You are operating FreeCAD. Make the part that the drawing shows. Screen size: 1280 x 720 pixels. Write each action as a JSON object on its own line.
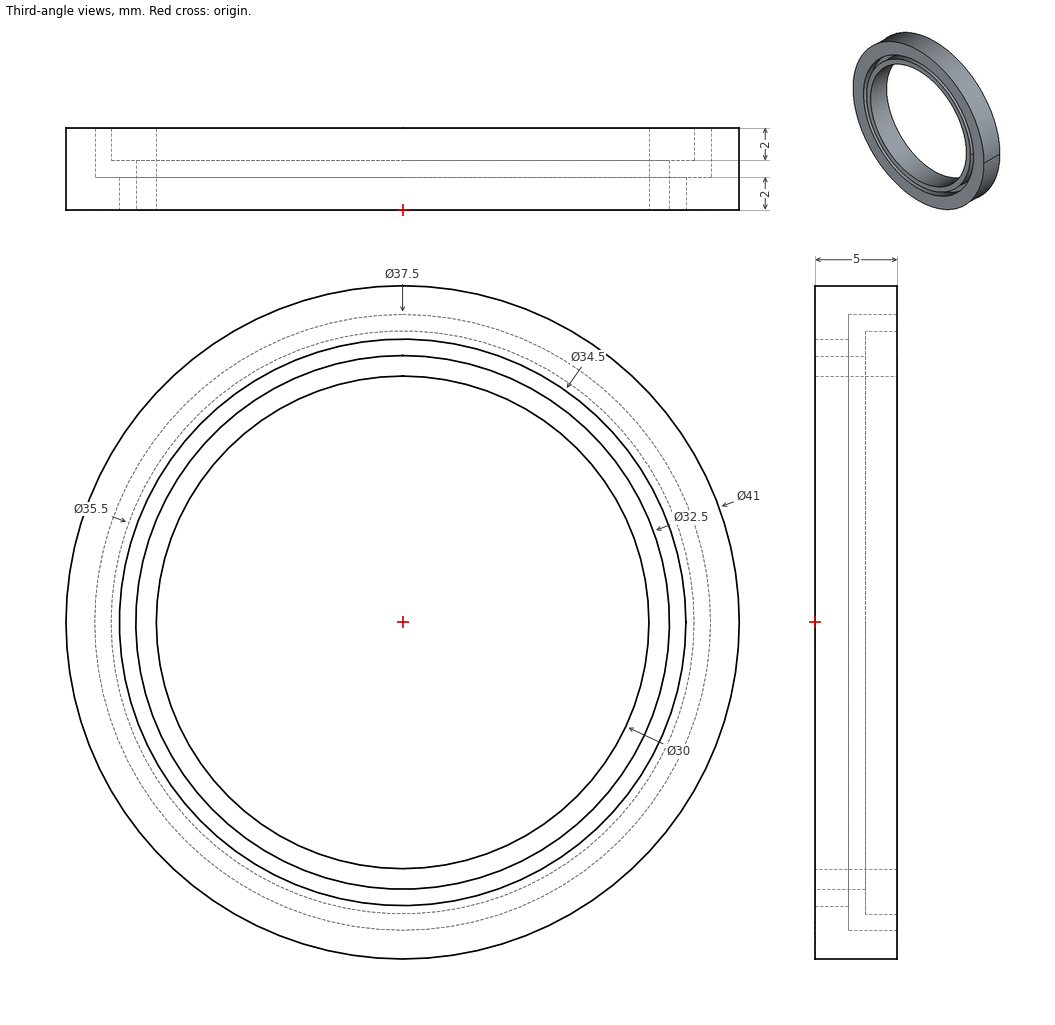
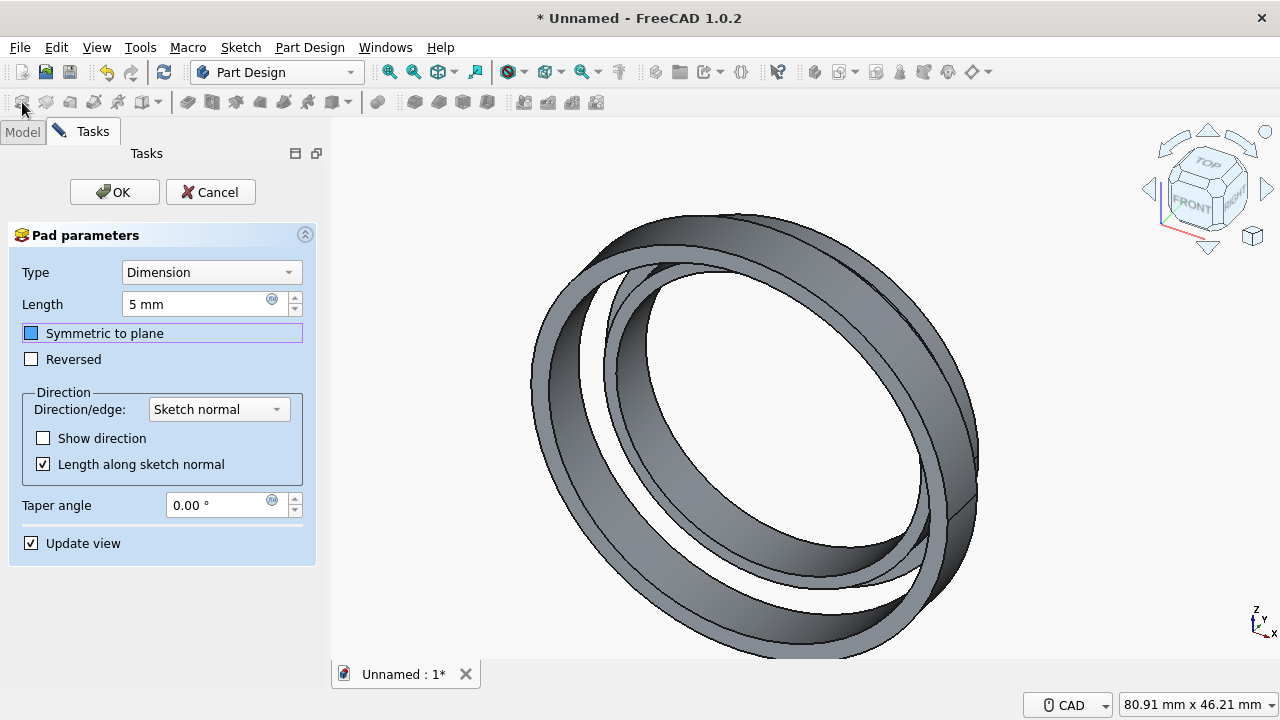
{"action": "left_click", "coordinate": [30, 359]}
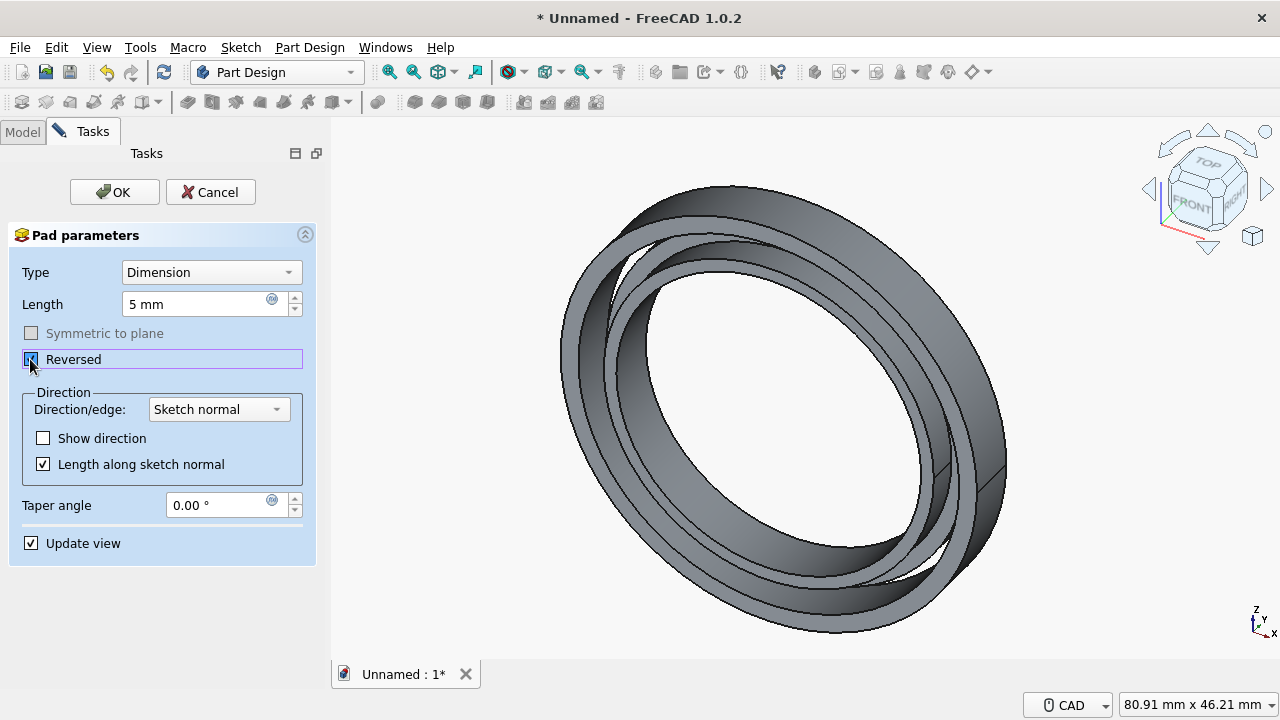
{"action": "left_click", "coordinate": [115, 192]}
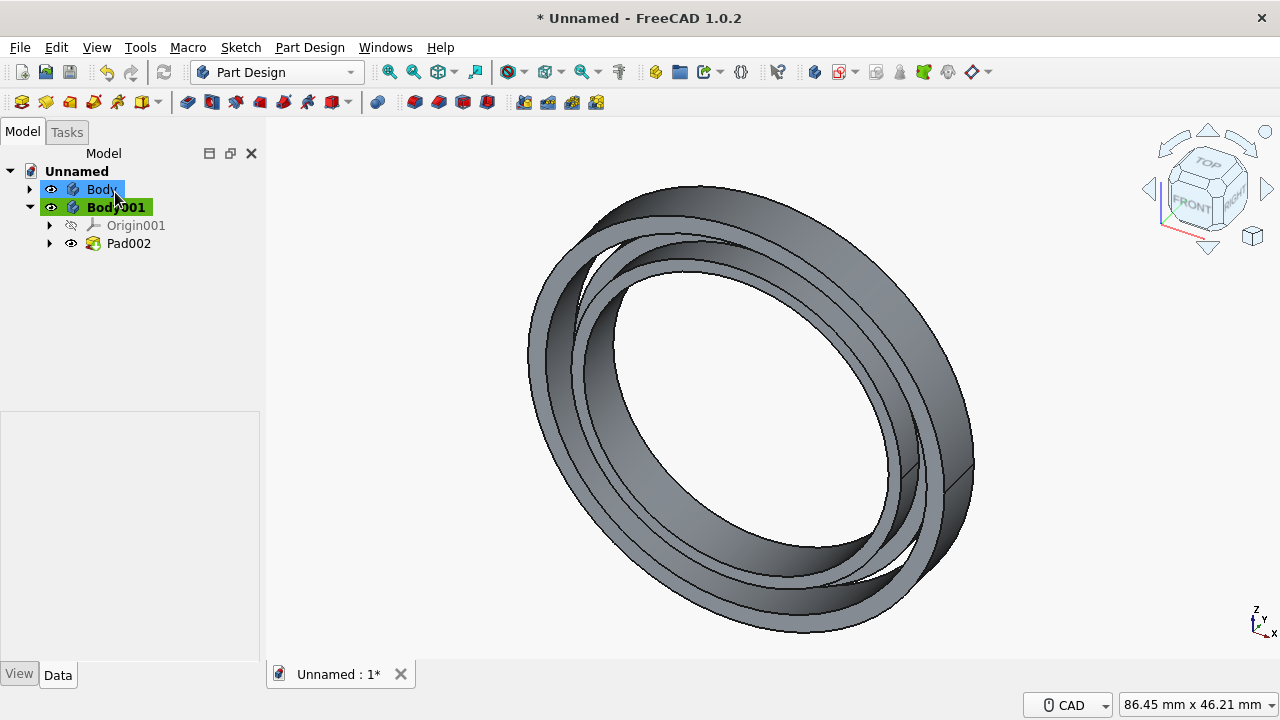
{"action": "left_click", "coordinate": [390, 72]}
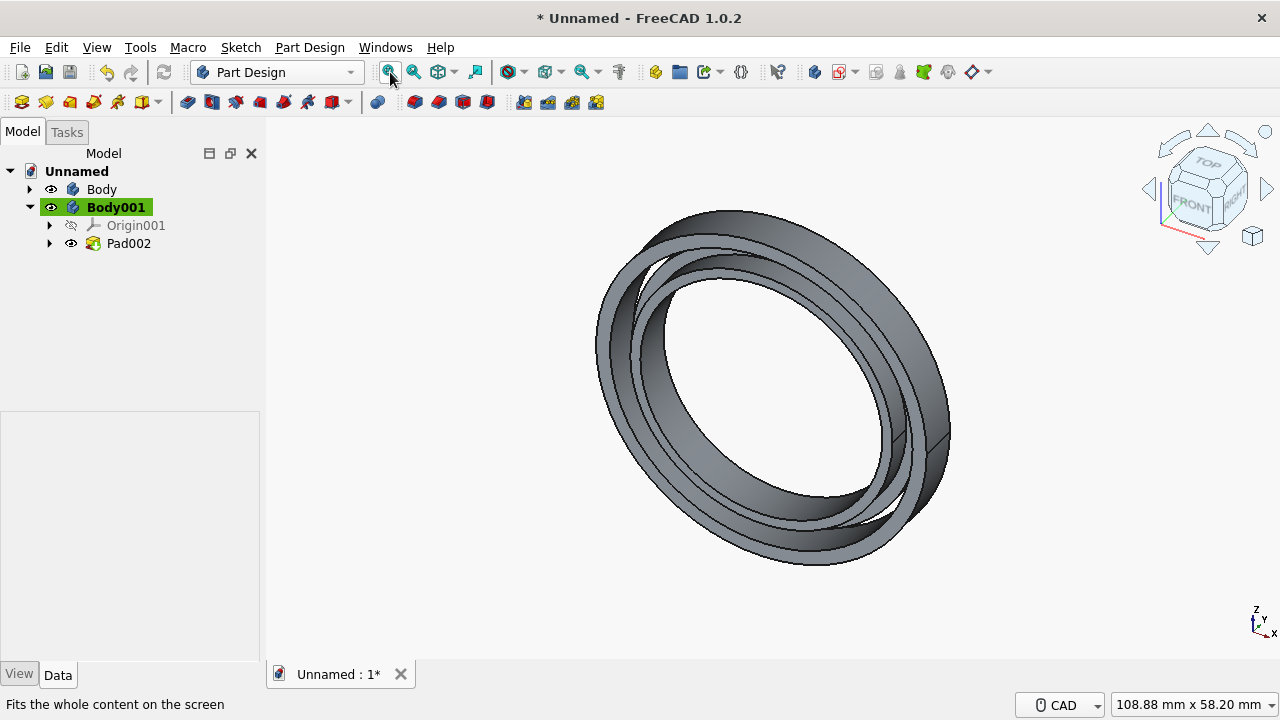
{"action": "left_click", "coordinate": [610, 299]}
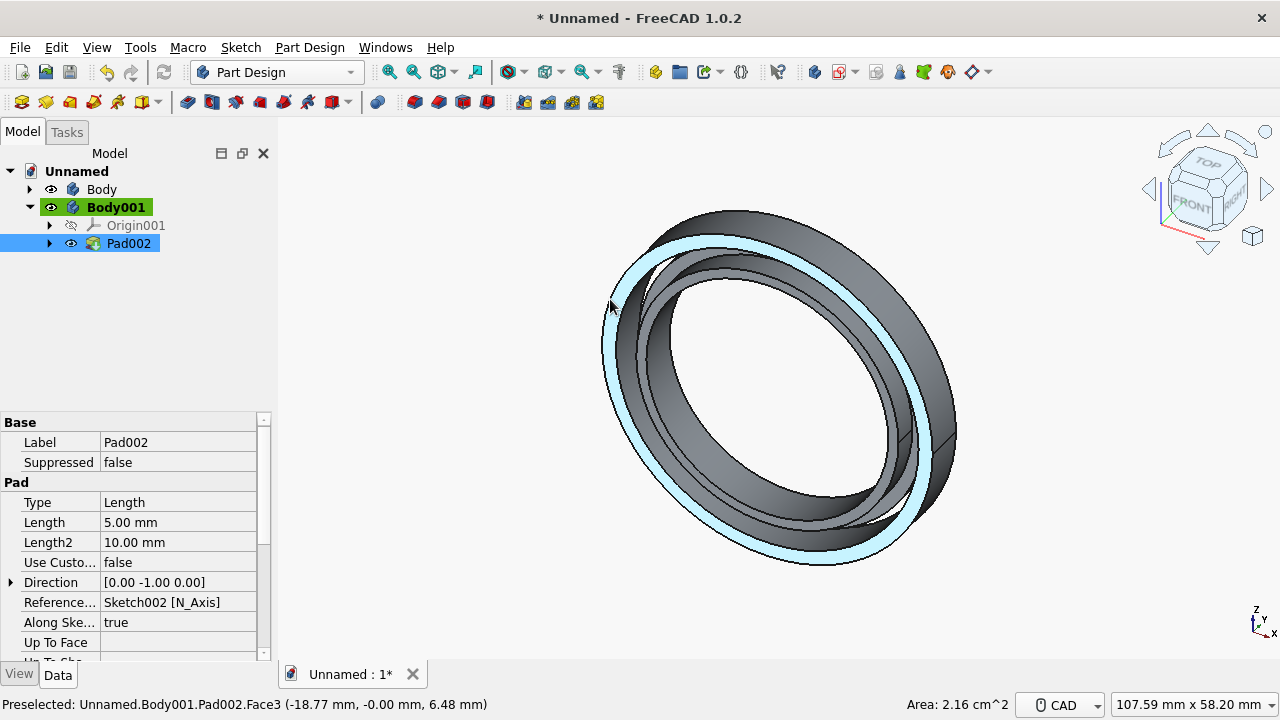
{"action": "left_click", "coordinate": [840, 72]}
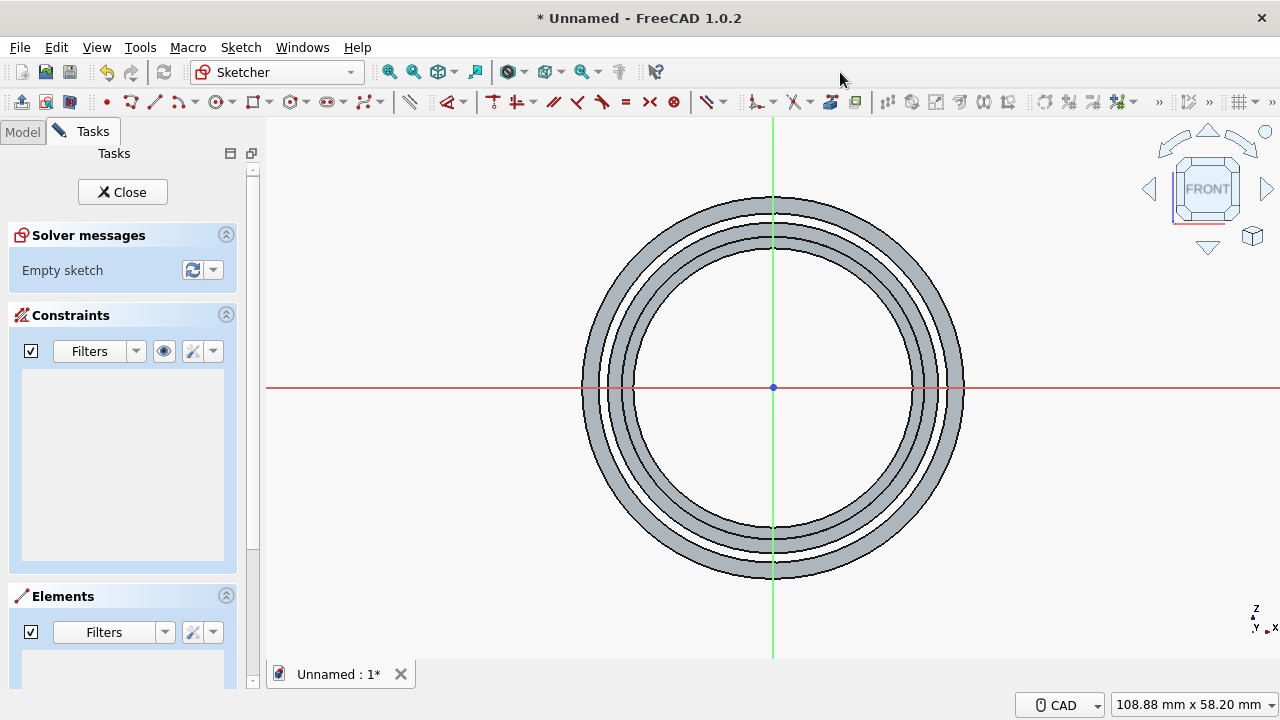
{"action": "left_click", "coordinate": [216, 102]}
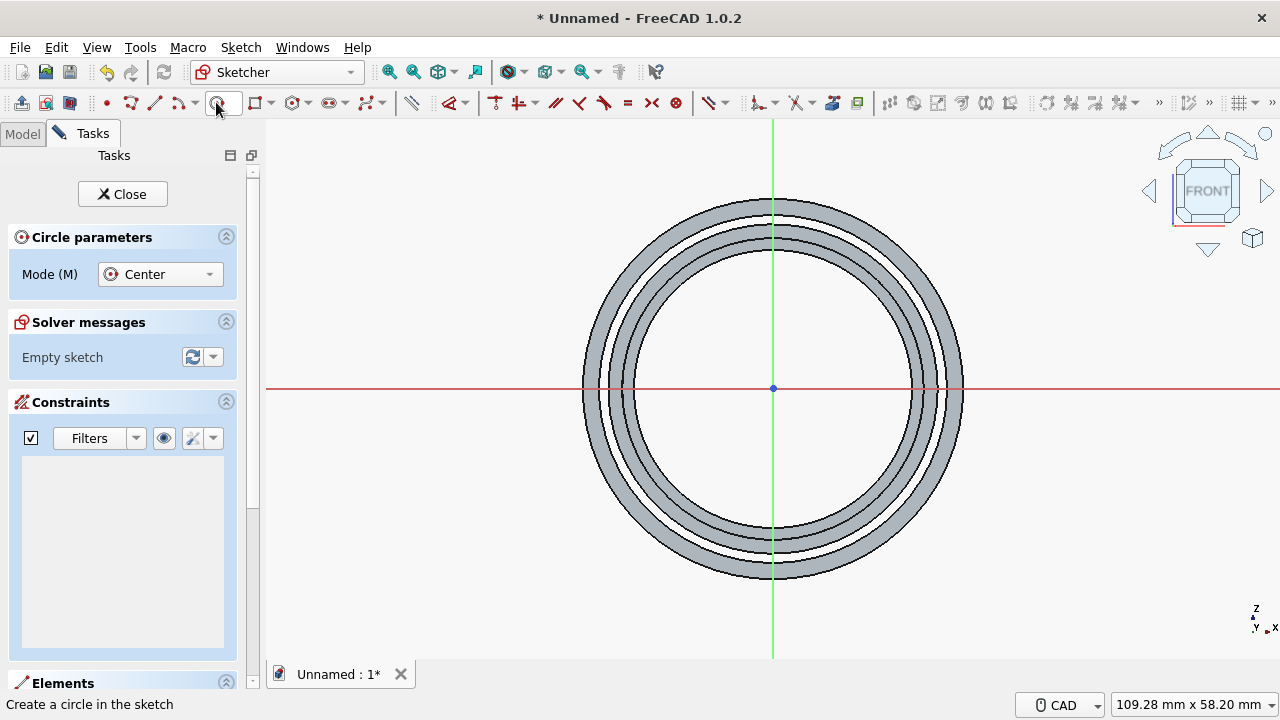
{"action": "left_click", "coordinate": [773, 389]}
{"action": "mouse_move", "coordinate": [896, 266]}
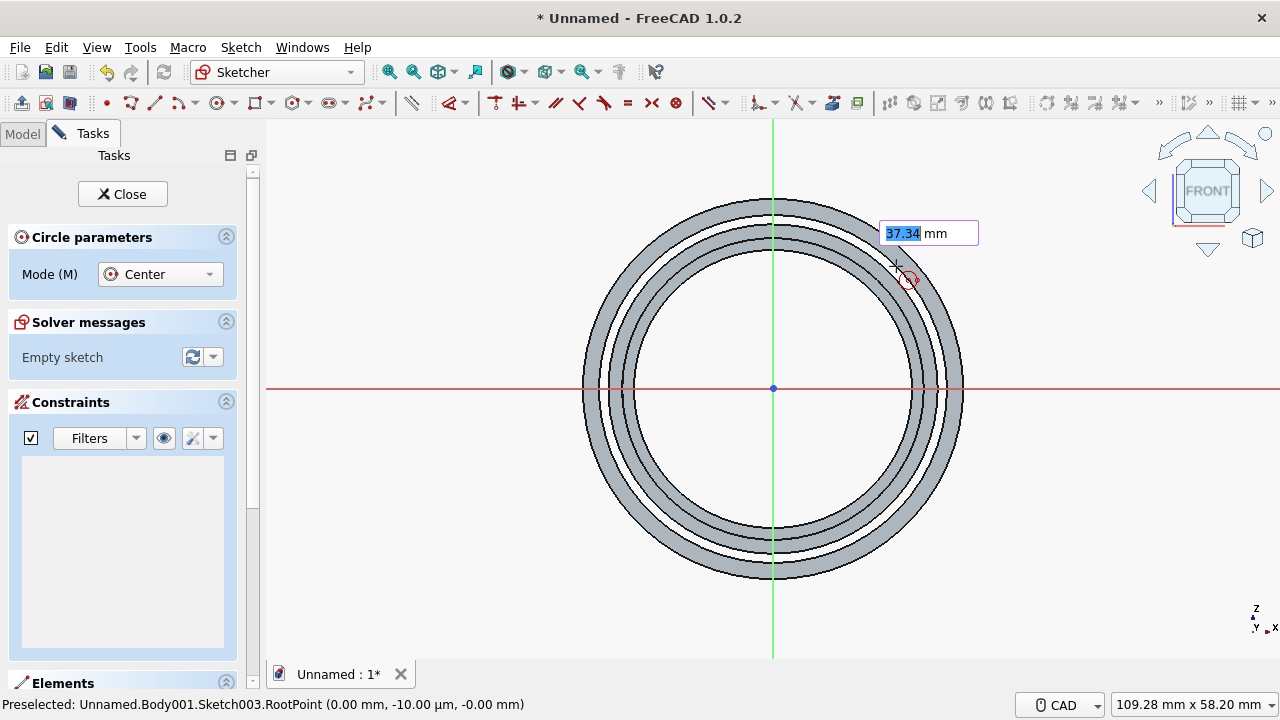
{"action": "type", "text": "37.5"}
{"action": "key", "text": "Return"}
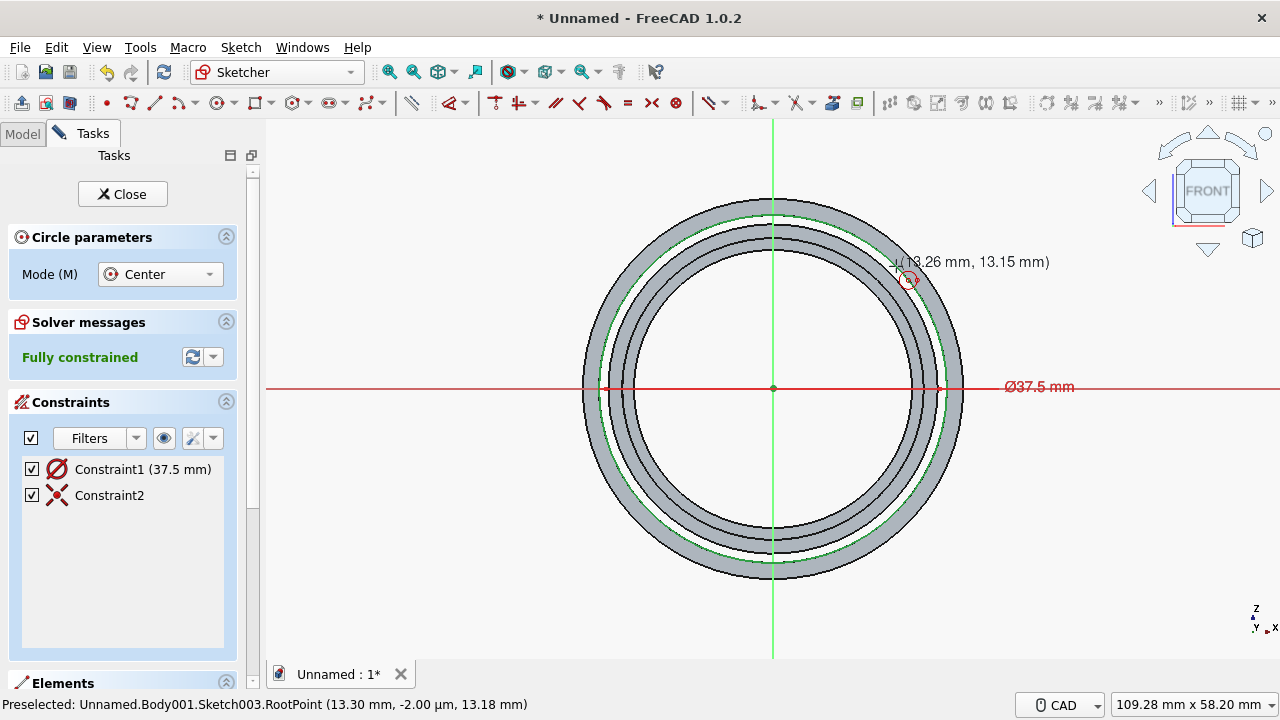
{"action": "left_click", "coordinate": [773, 389]}
{"action": "mouse_move", "coordinate": [886, 276]}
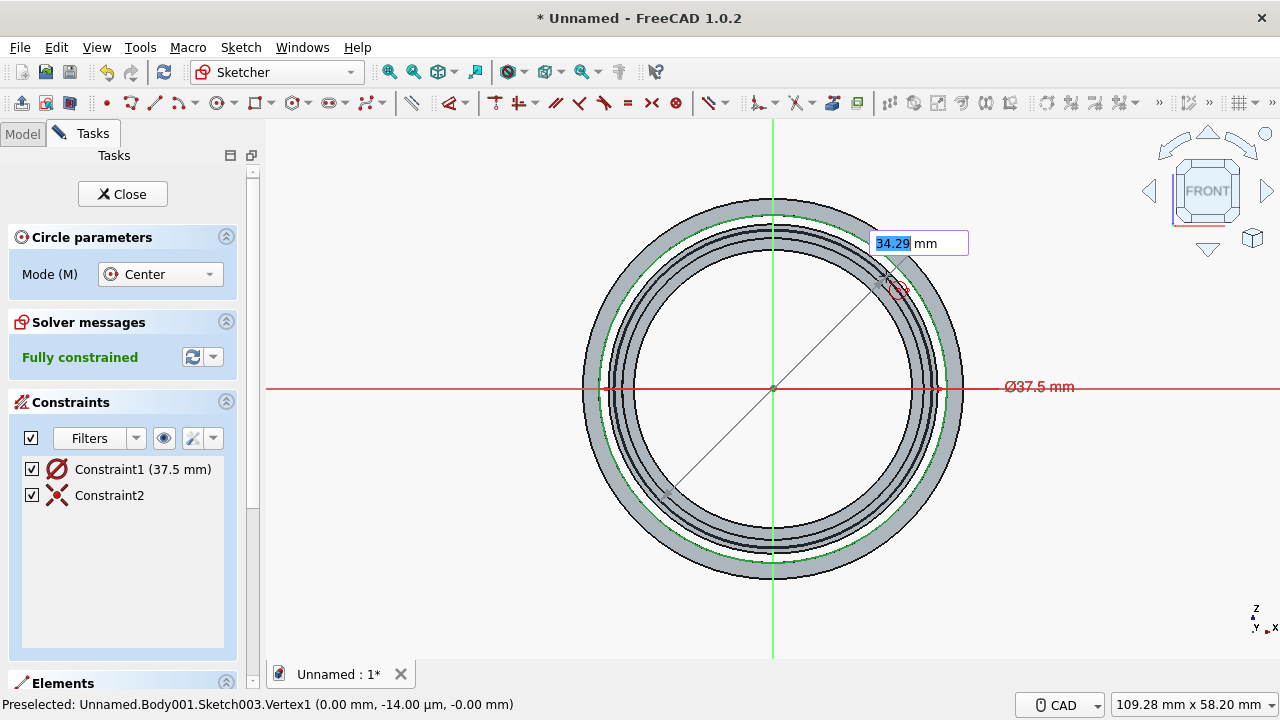
{"action": "type", "text": "34.5"}
{"action": "key", "text": "Return"}
{"action": "key", "text": "Escape"}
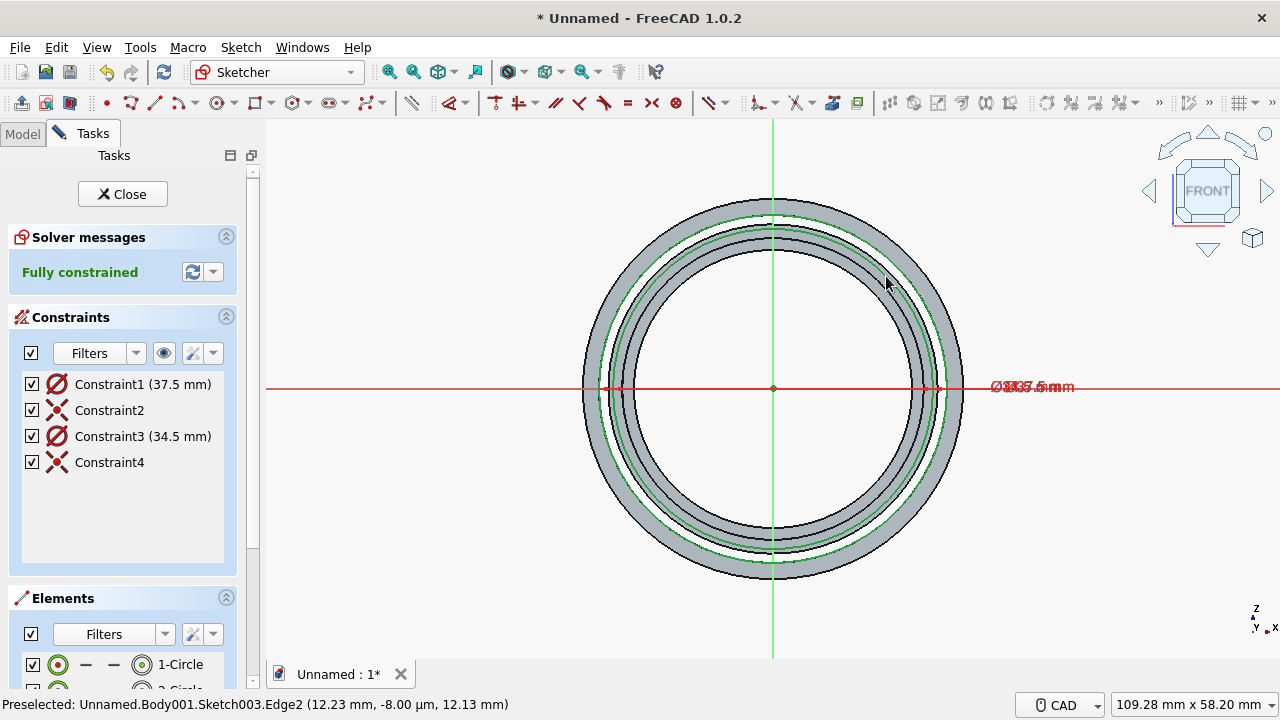
{"action": "left_click", "coordinate": [123, 194]}